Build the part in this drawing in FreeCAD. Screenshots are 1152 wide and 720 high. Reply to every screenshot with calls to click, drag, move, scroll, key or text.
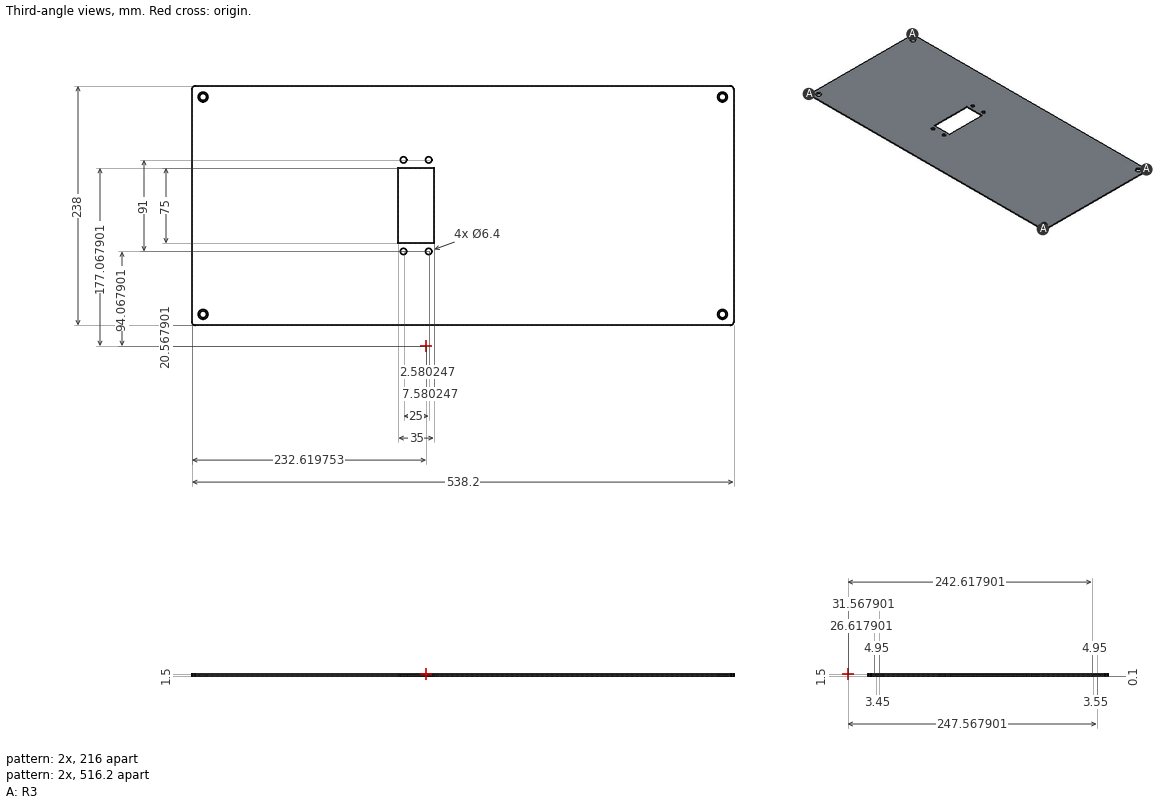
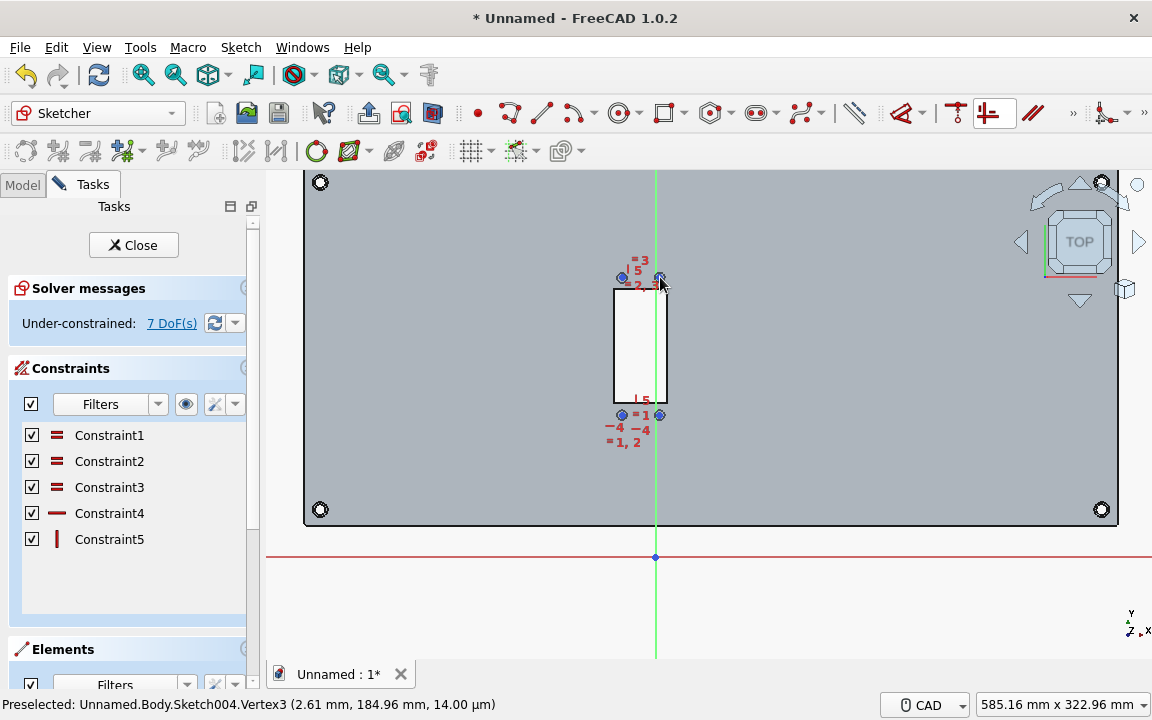
click(622, 415)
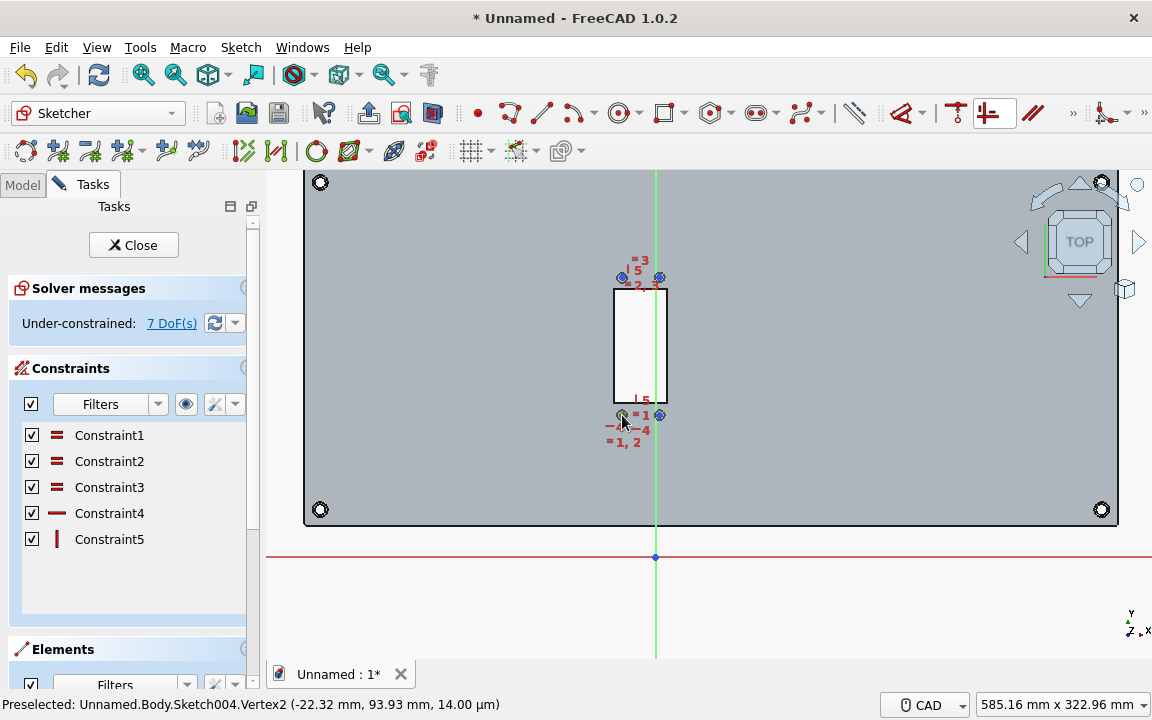
click(620, 280)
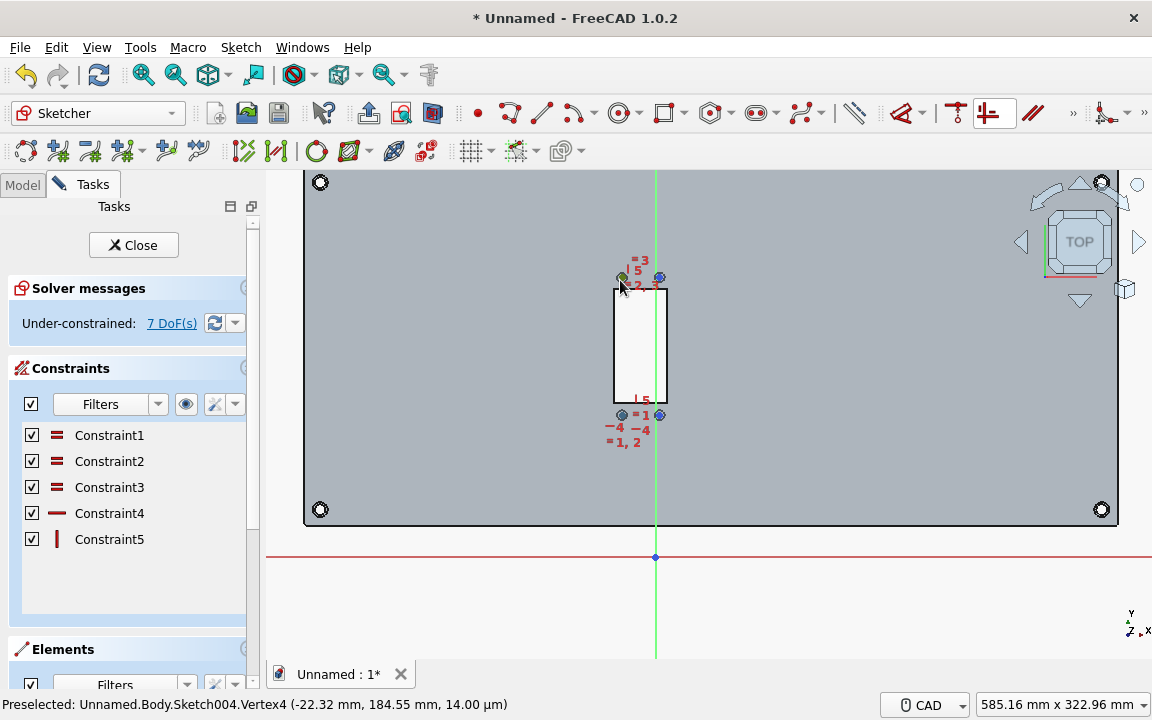
key(v)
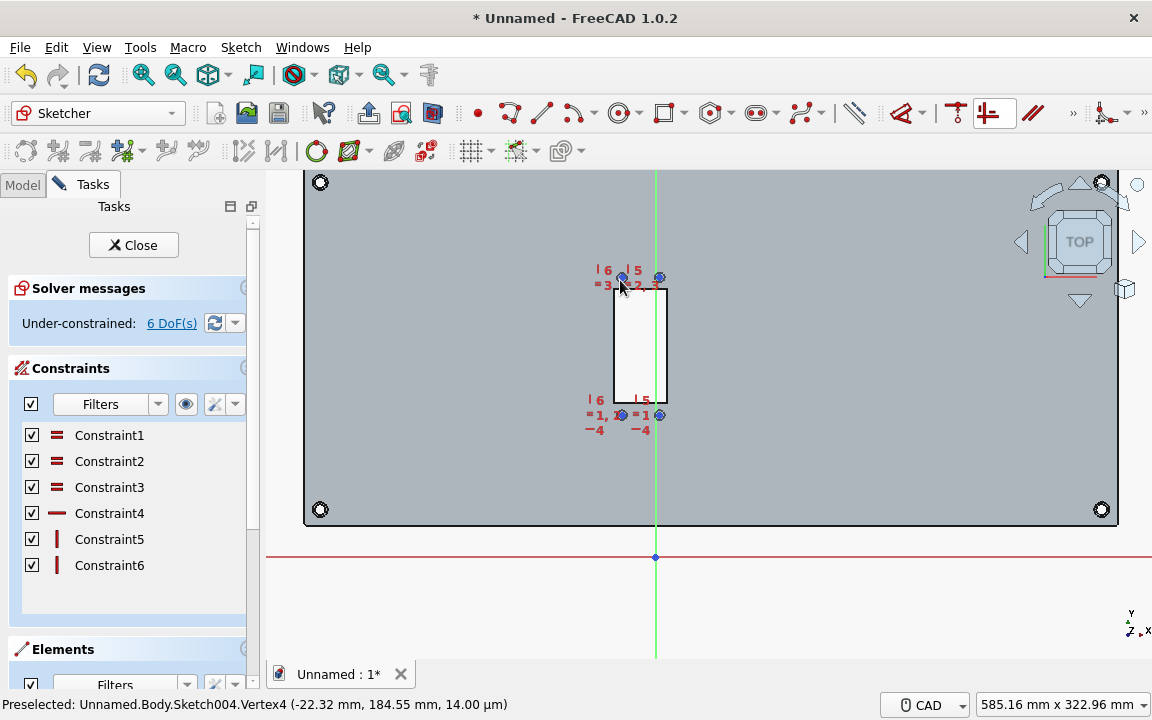
click(660, 277)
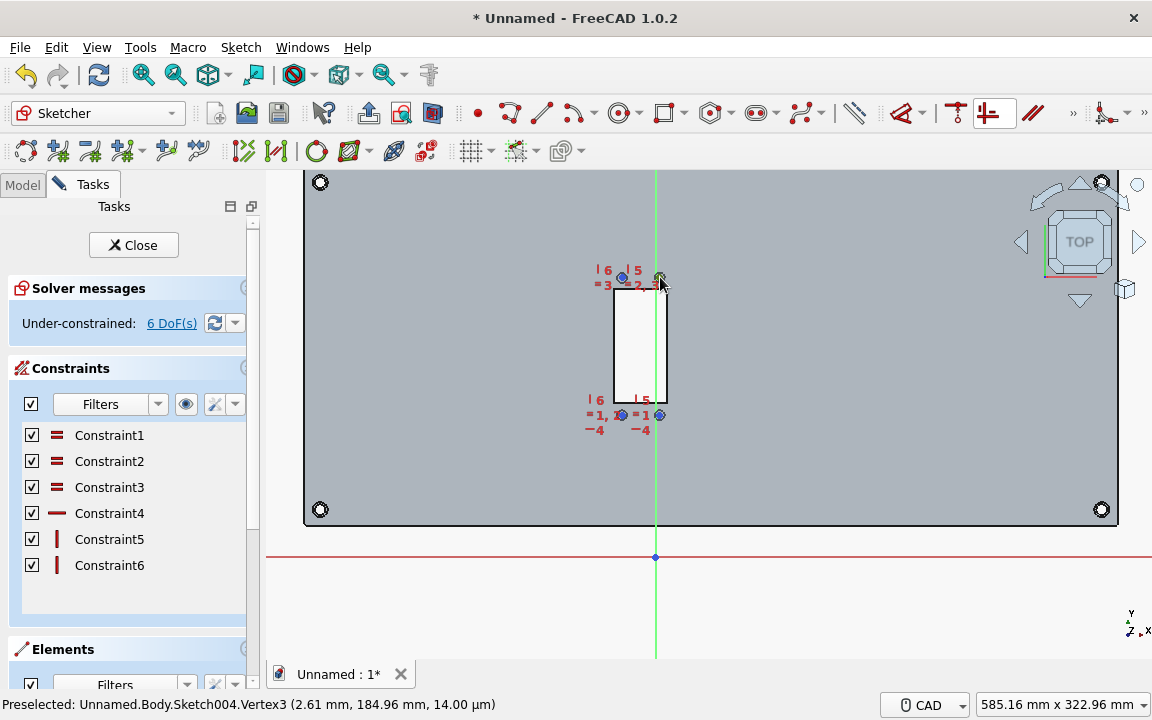
click(620, 280)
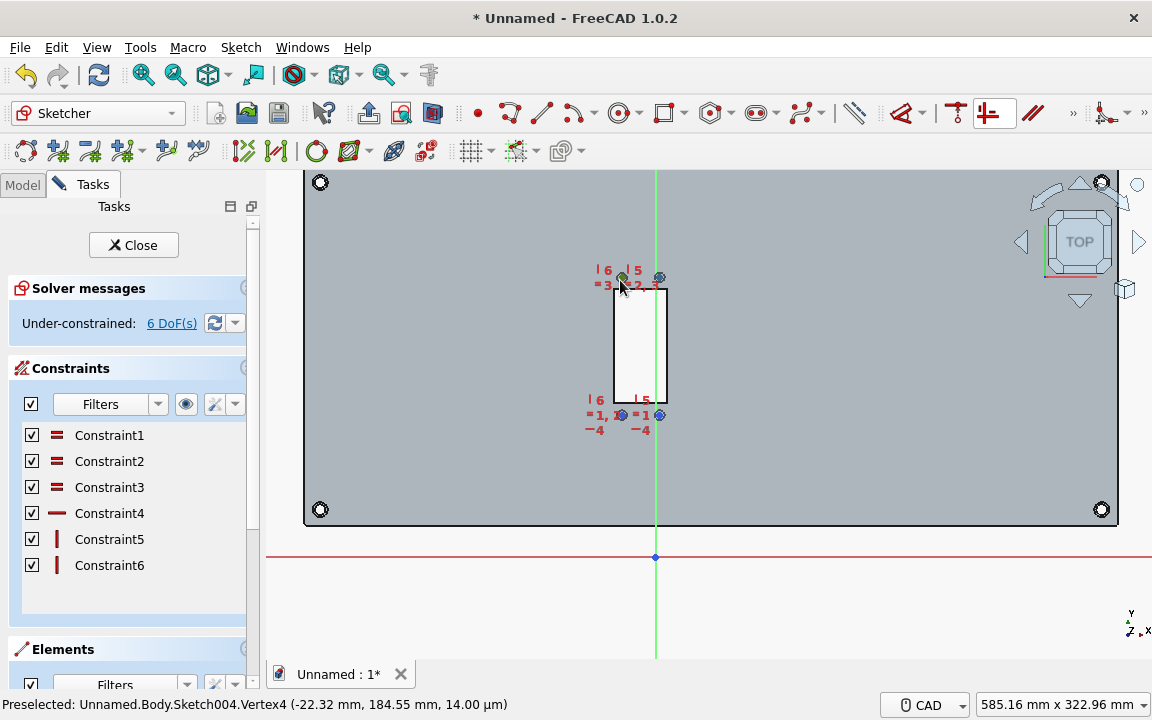
key(h)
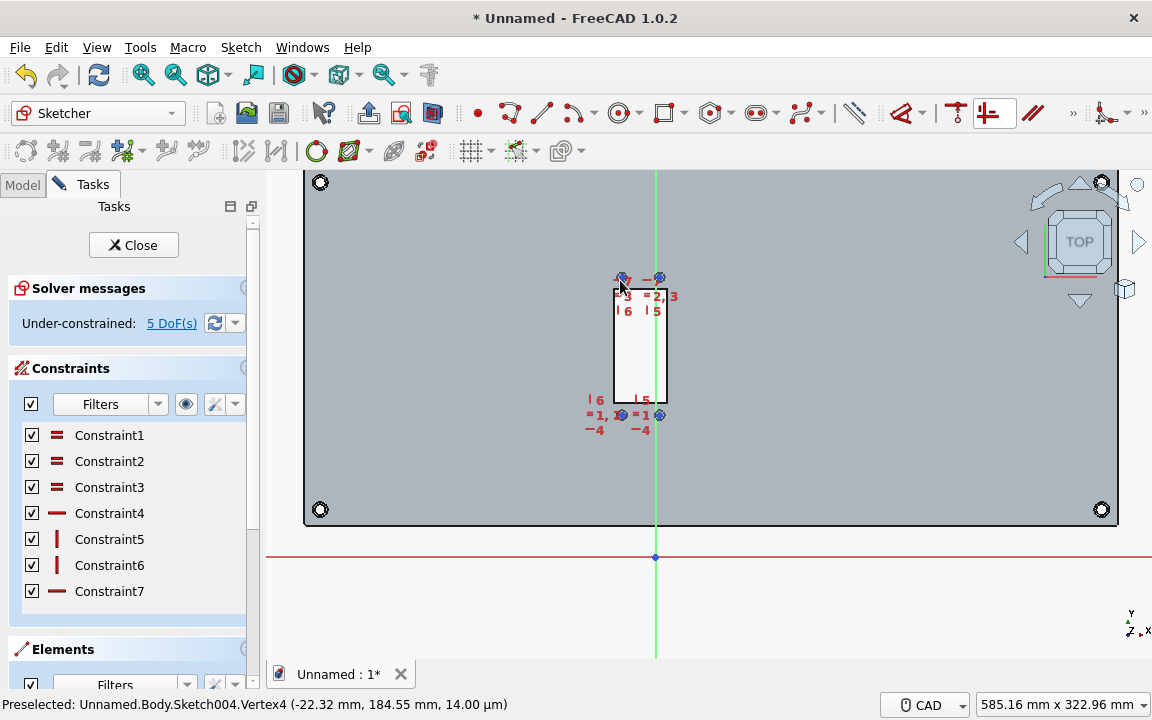
click(902, 114)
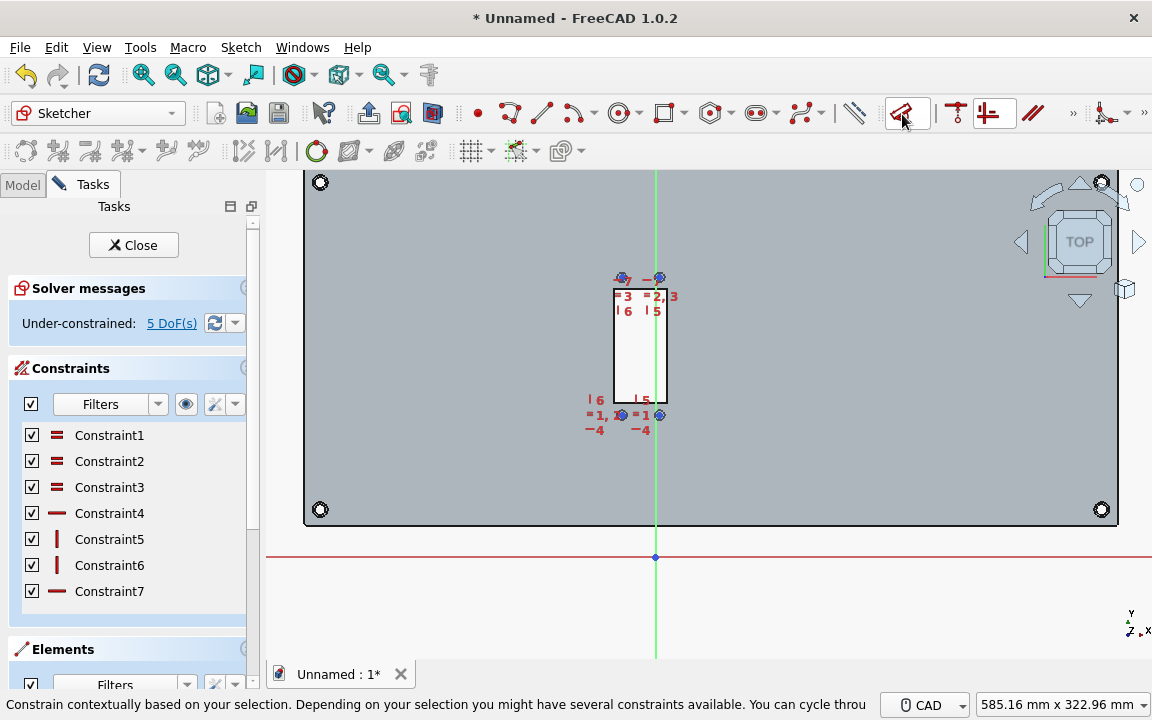
scroll(660, 420, up, 8)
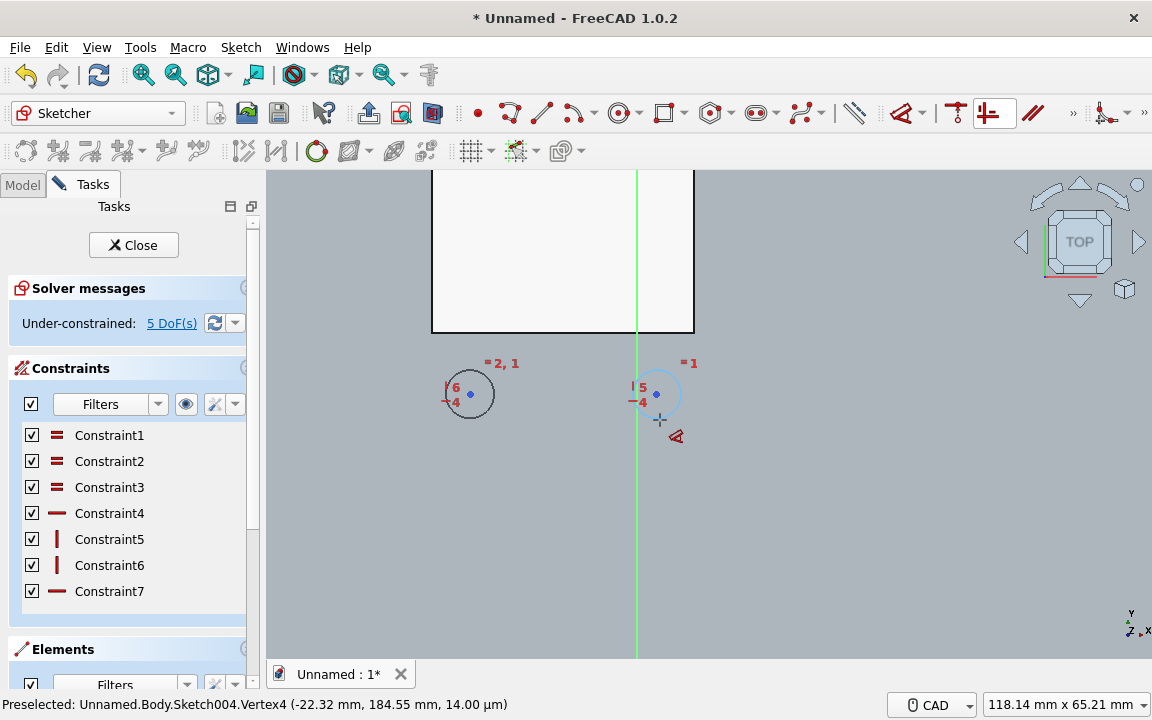
click(656, 418)
click(655, 450)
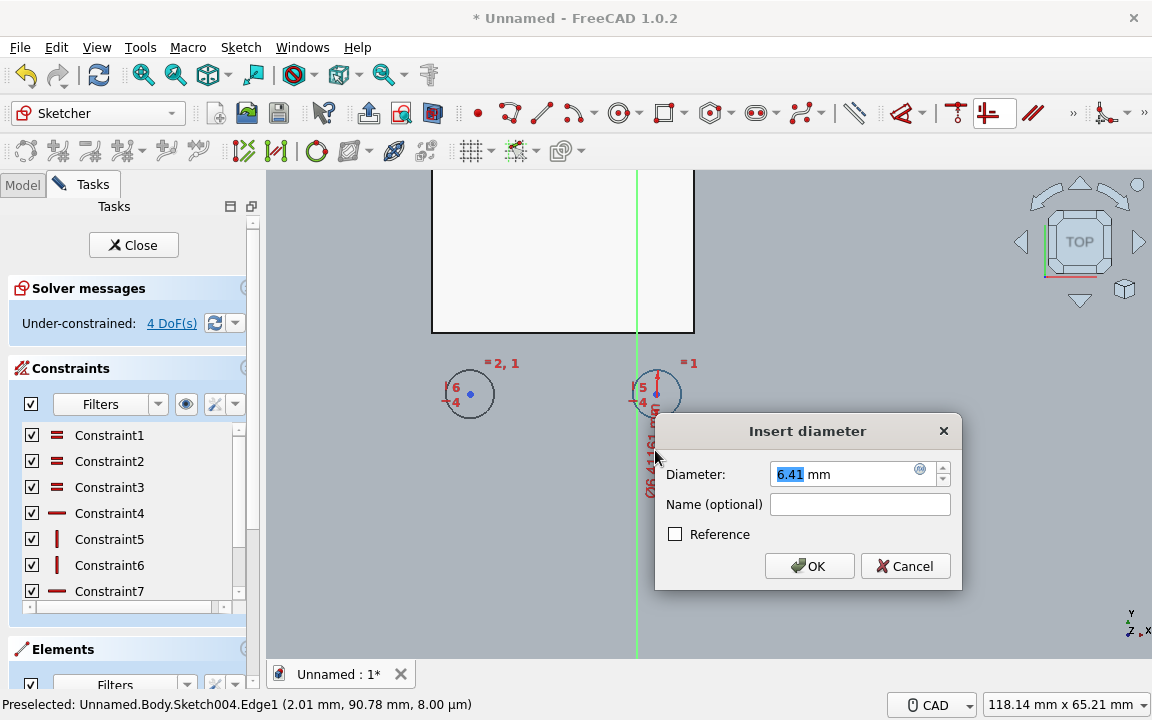
text(6.4)
key(Return)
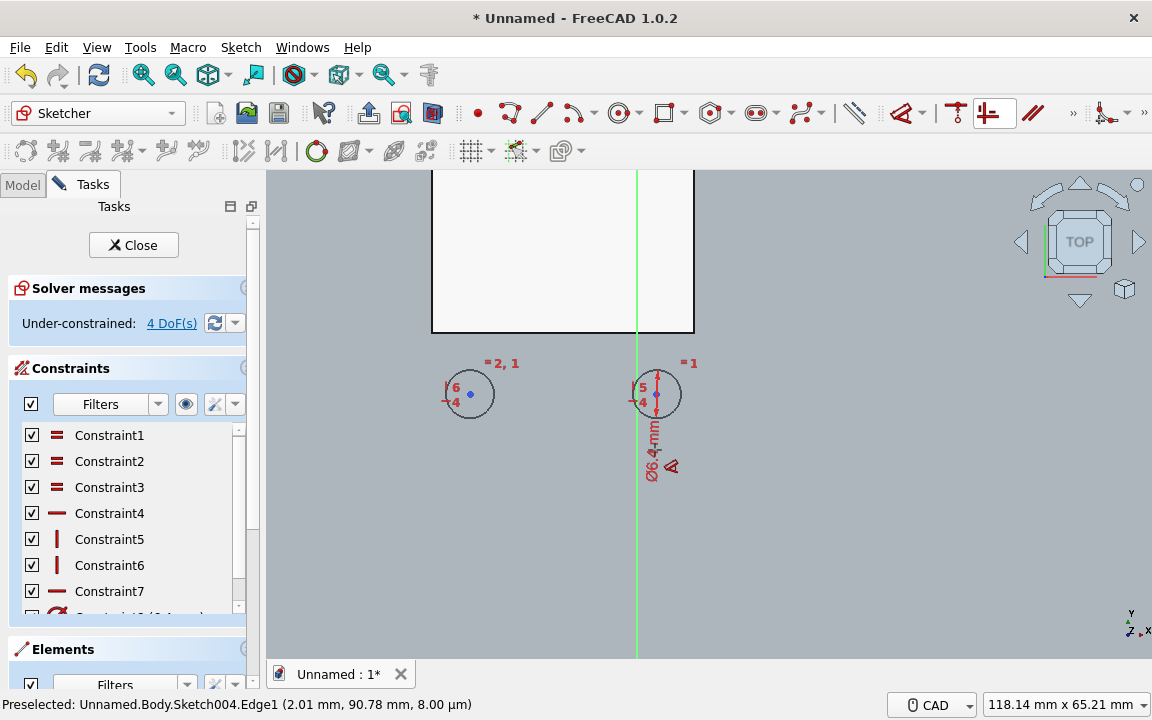
scroll(660, 420, down, 8)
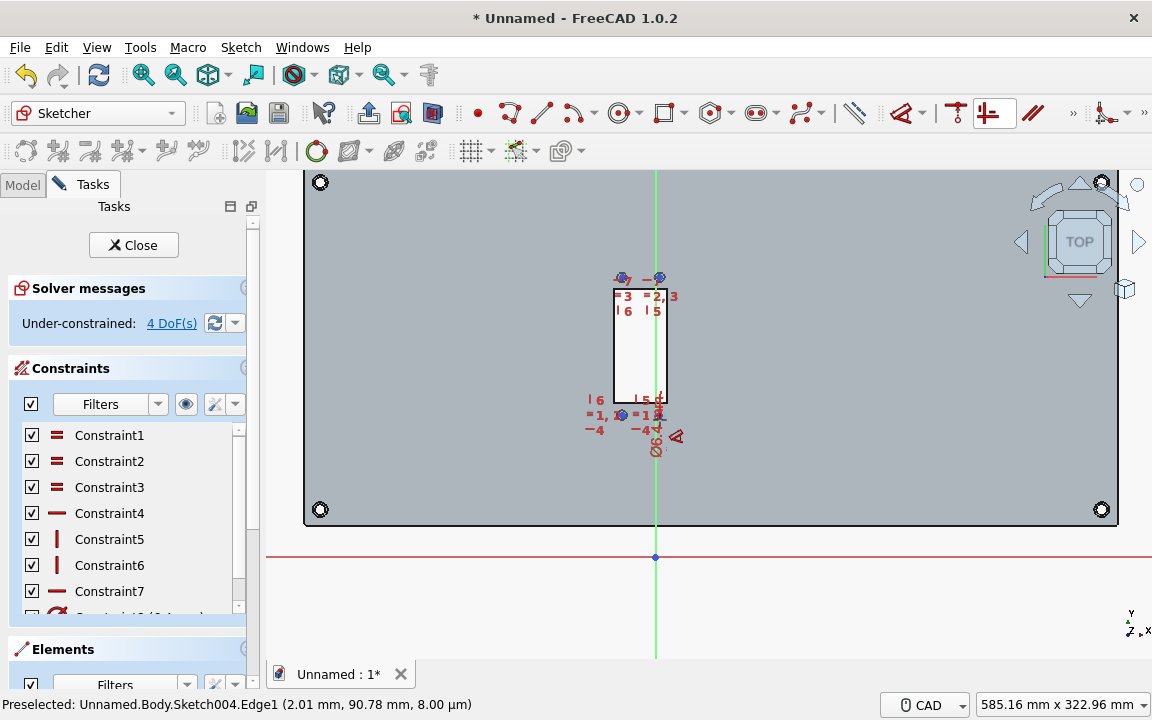
click(660, 415)